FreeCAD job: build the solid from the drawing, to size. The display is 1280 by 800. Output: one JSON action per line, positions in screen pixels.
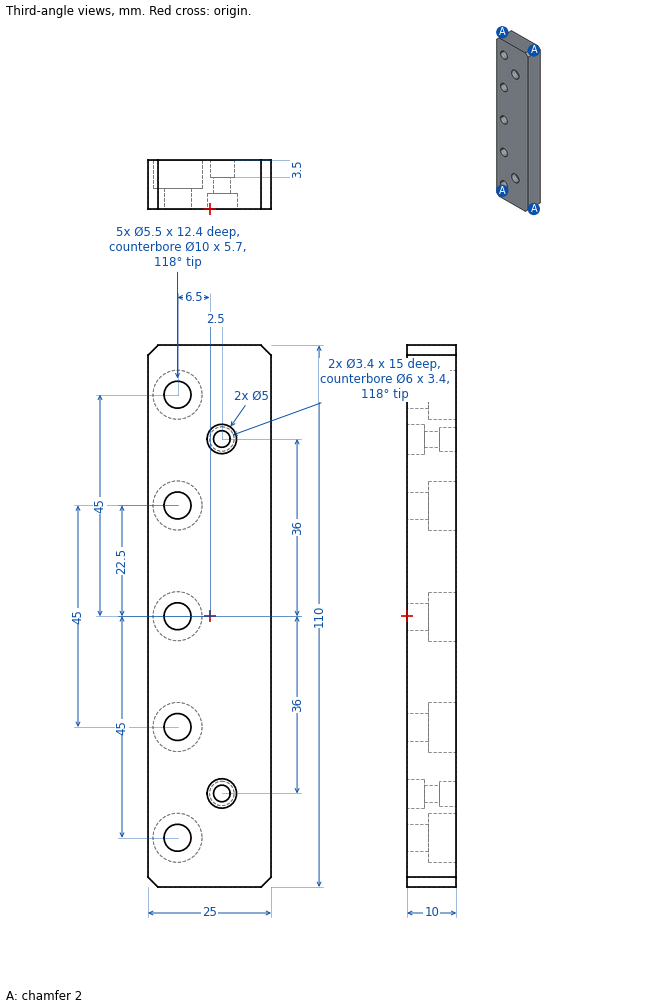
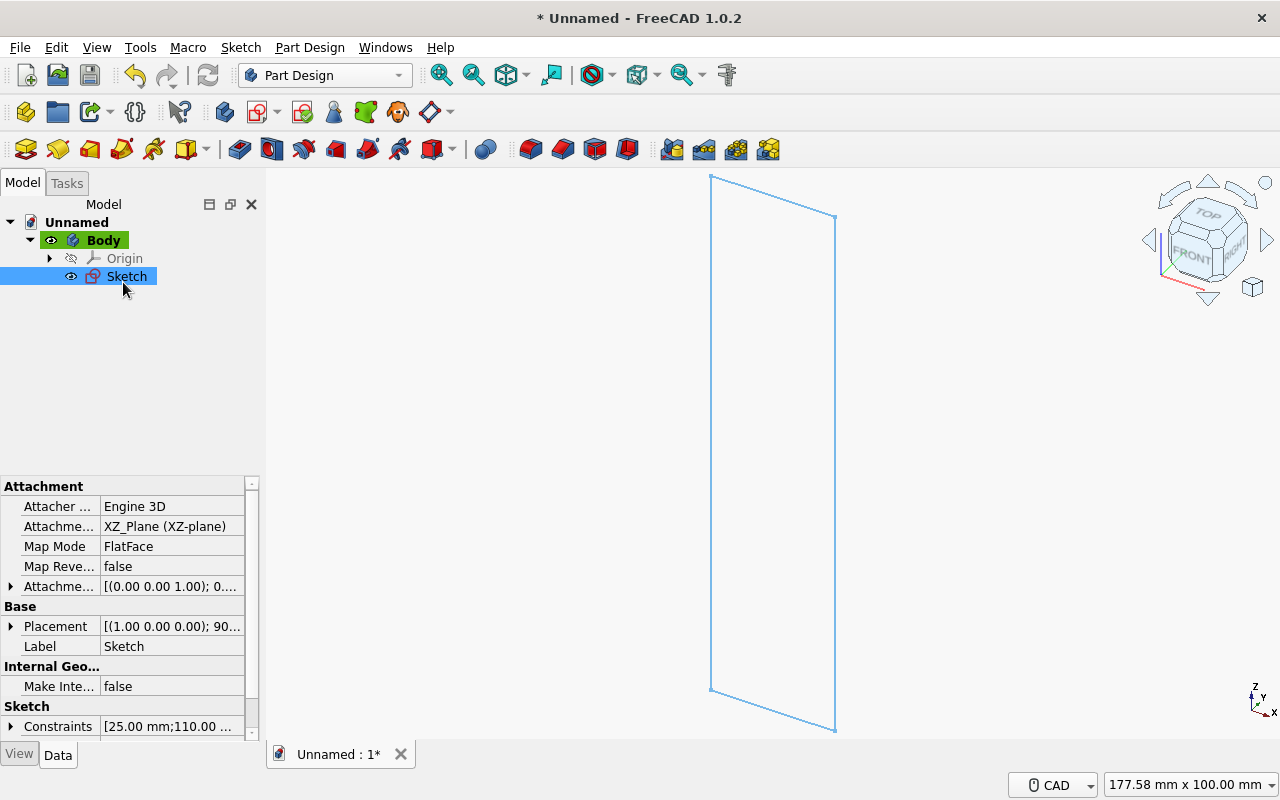
{"action": "left_click", "coordinate": [26, 150]}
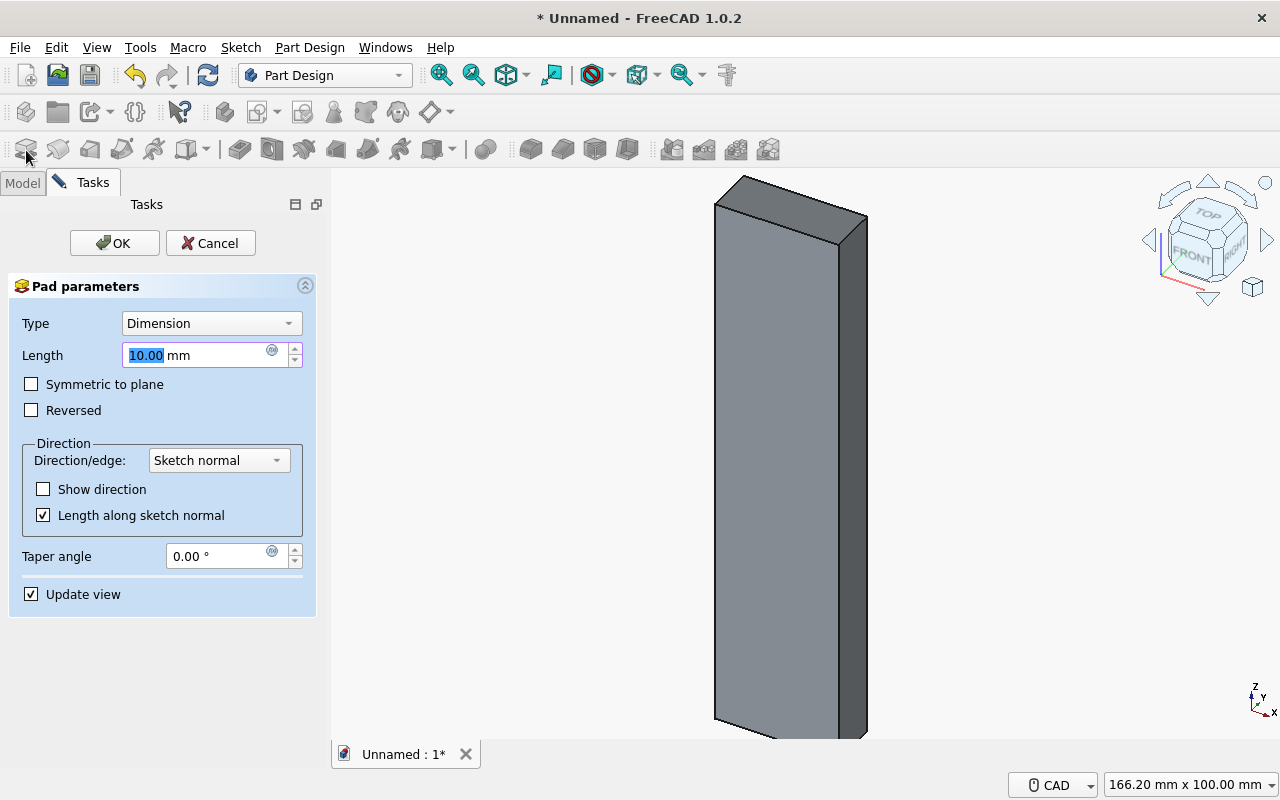
{"action": "type", "text": "10"}
{"action": "key", "text": "Tab"}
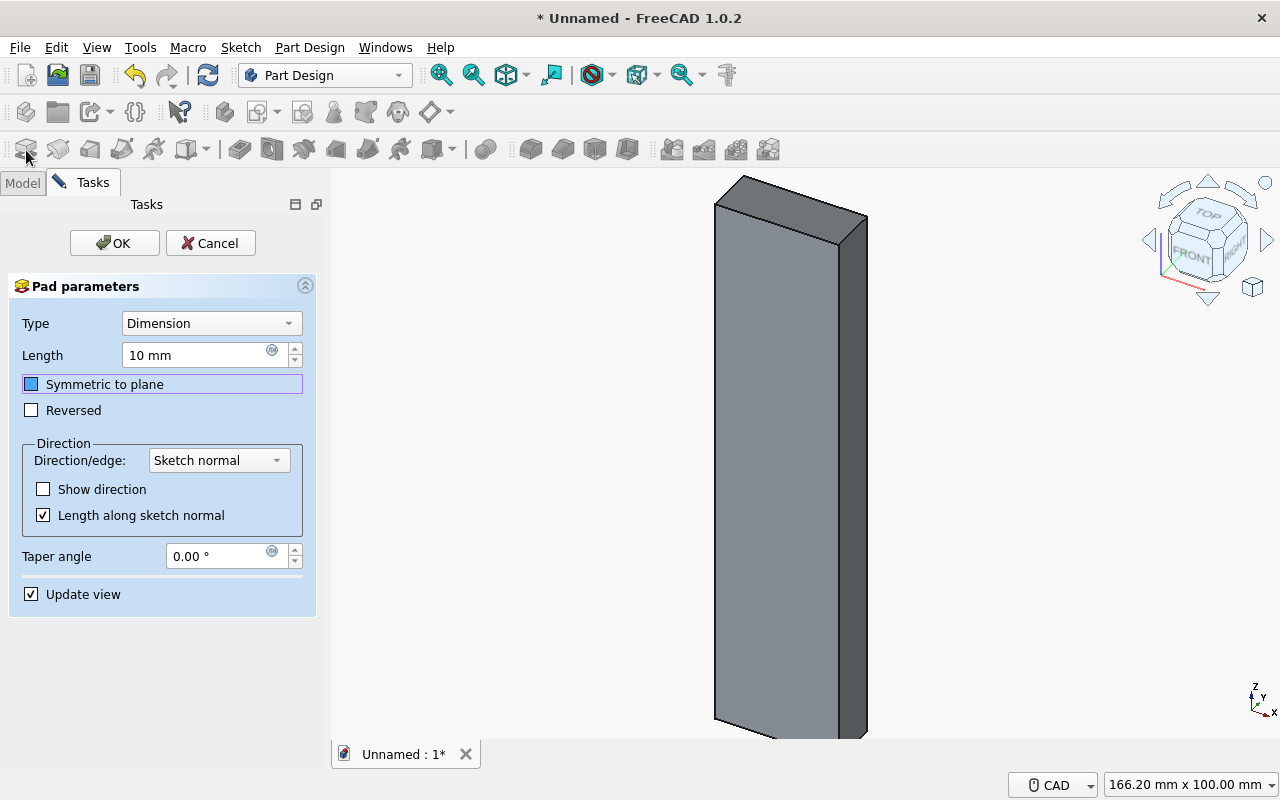
{"action": "left_click", "coordinate": [30, 410]}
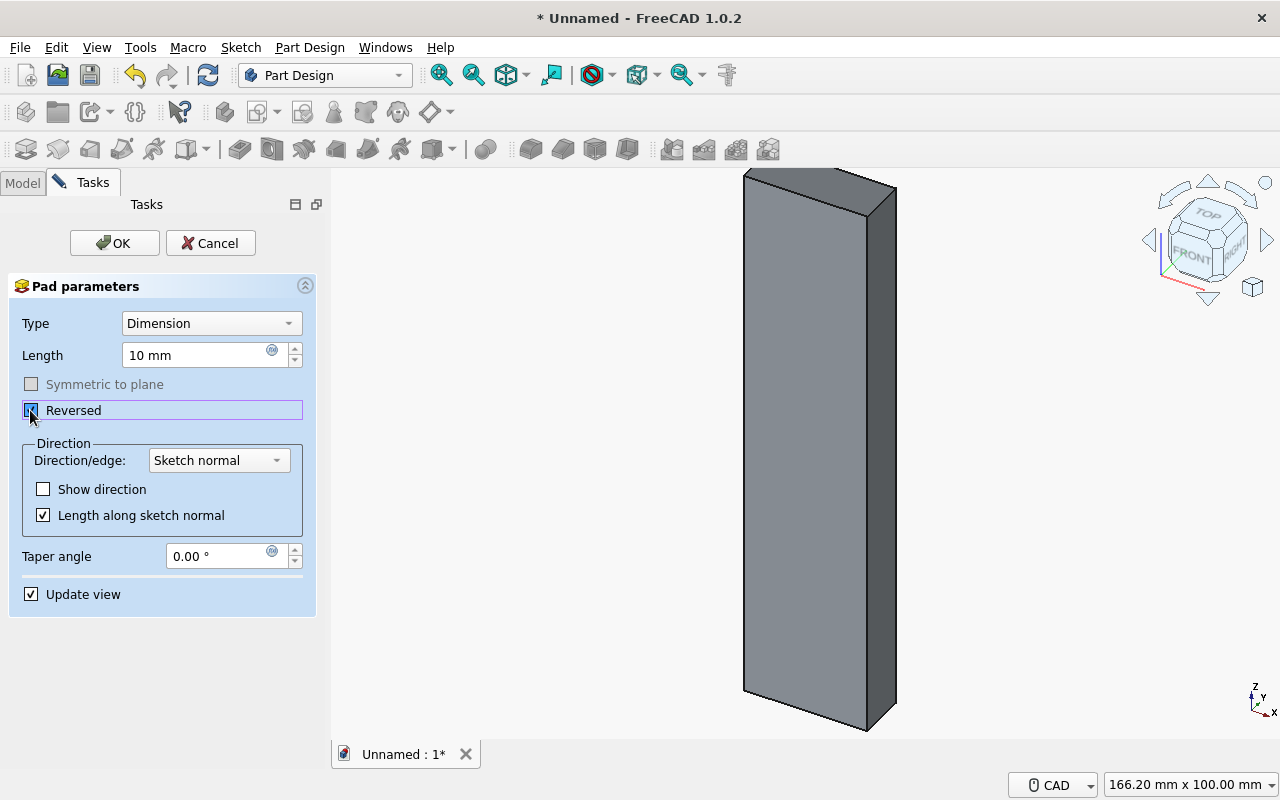
{"action": "left_click", "coordinate": [115, 243]}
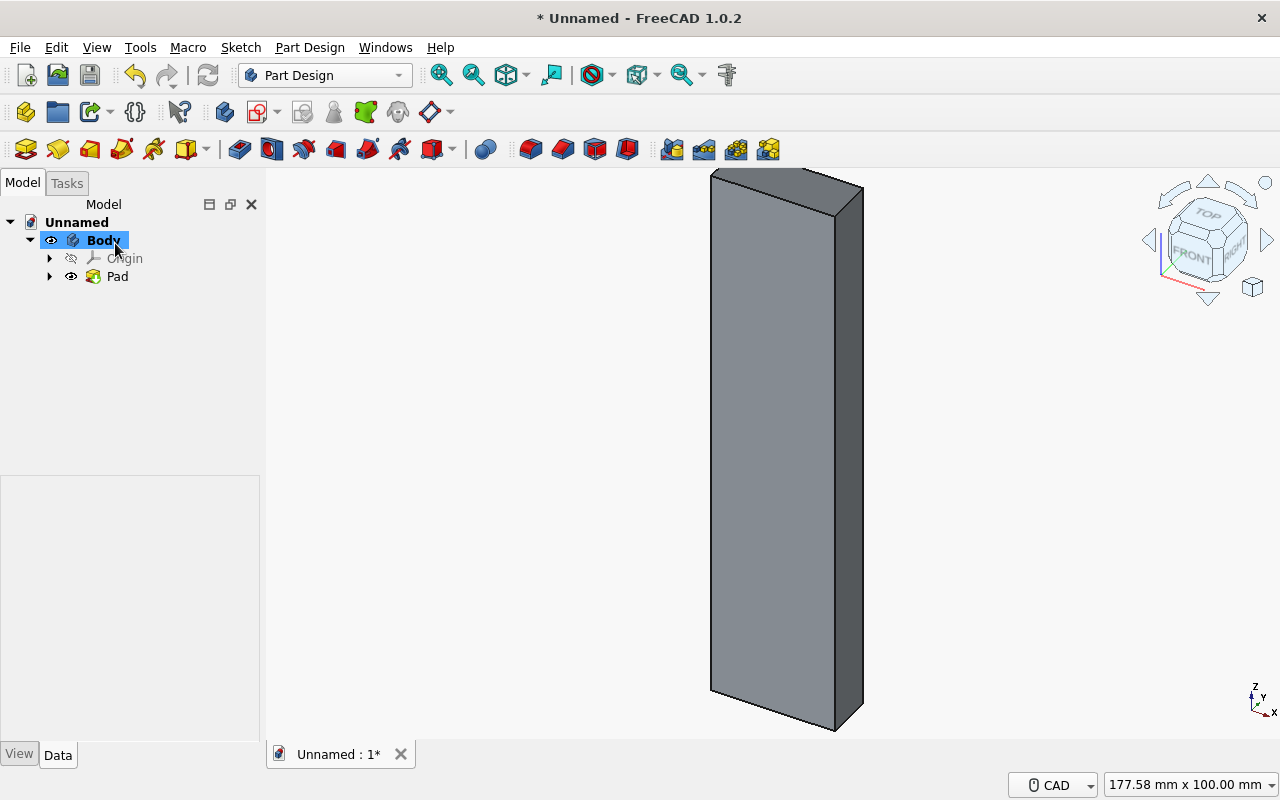
{"action": "left_click", "coordinate": [442, 76]}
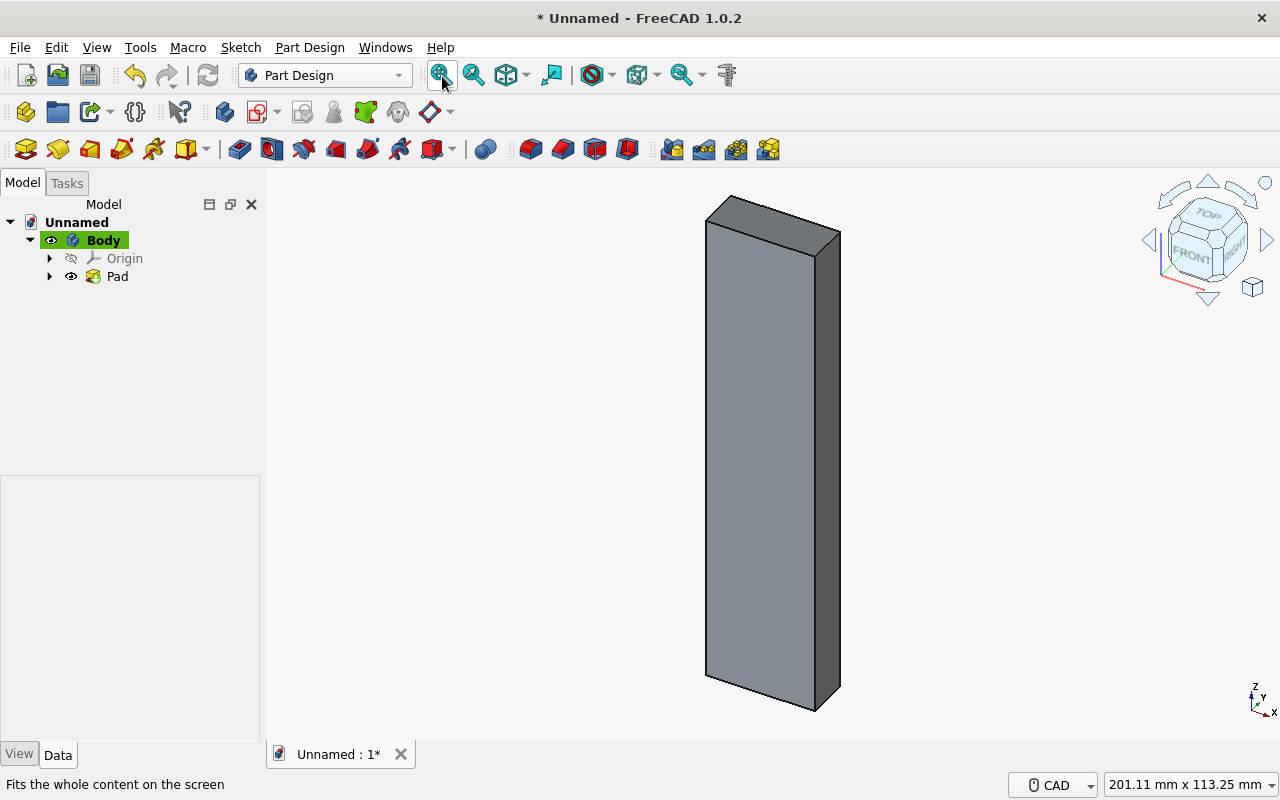
{"action": "left_click", "coordinate": [828, 243]}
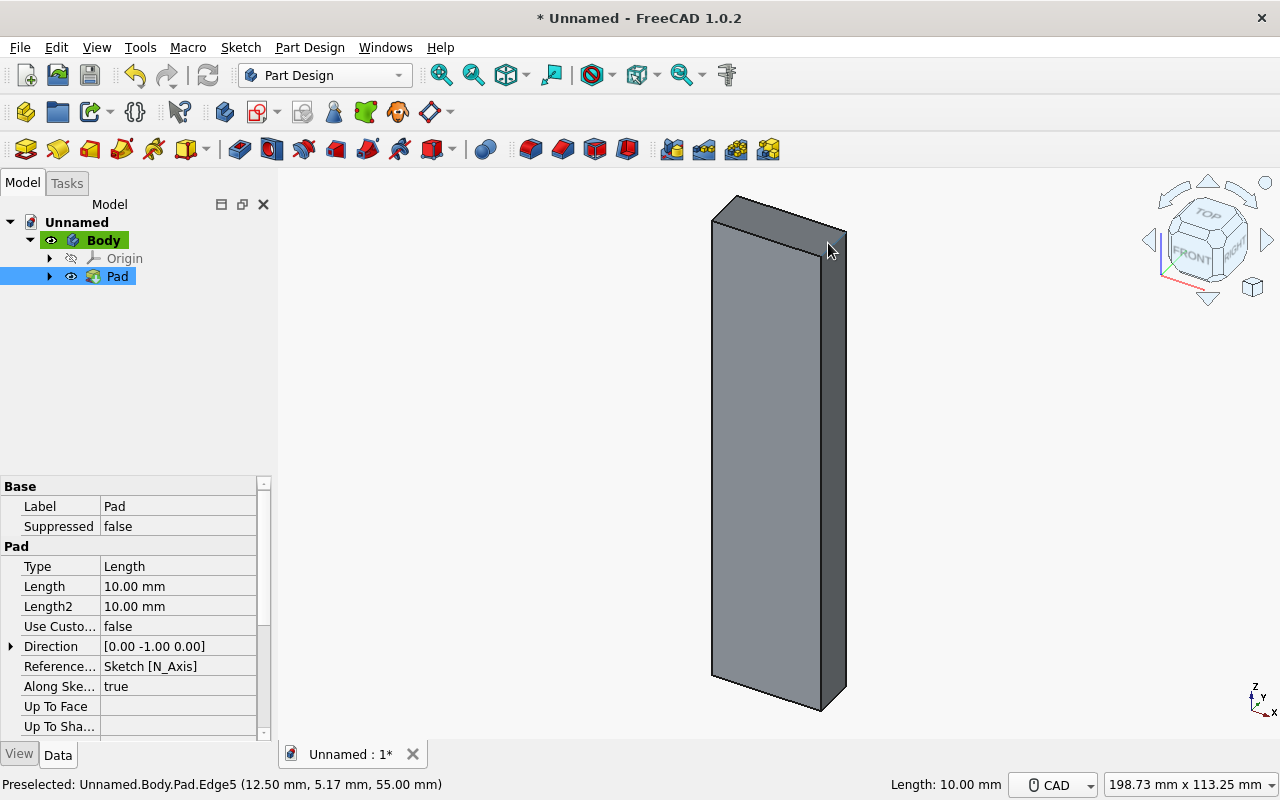
{"action": "key", "text": "0"}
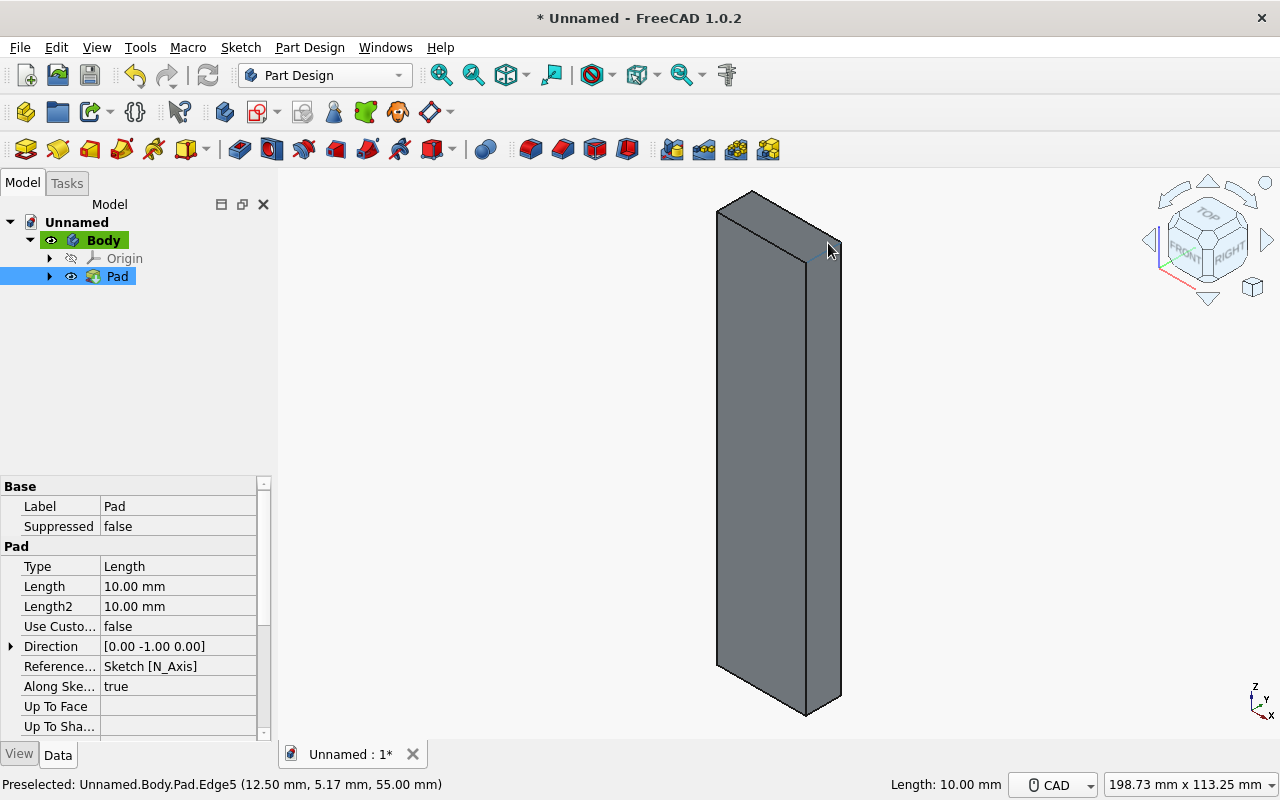
{"action": "key", "text": "2"}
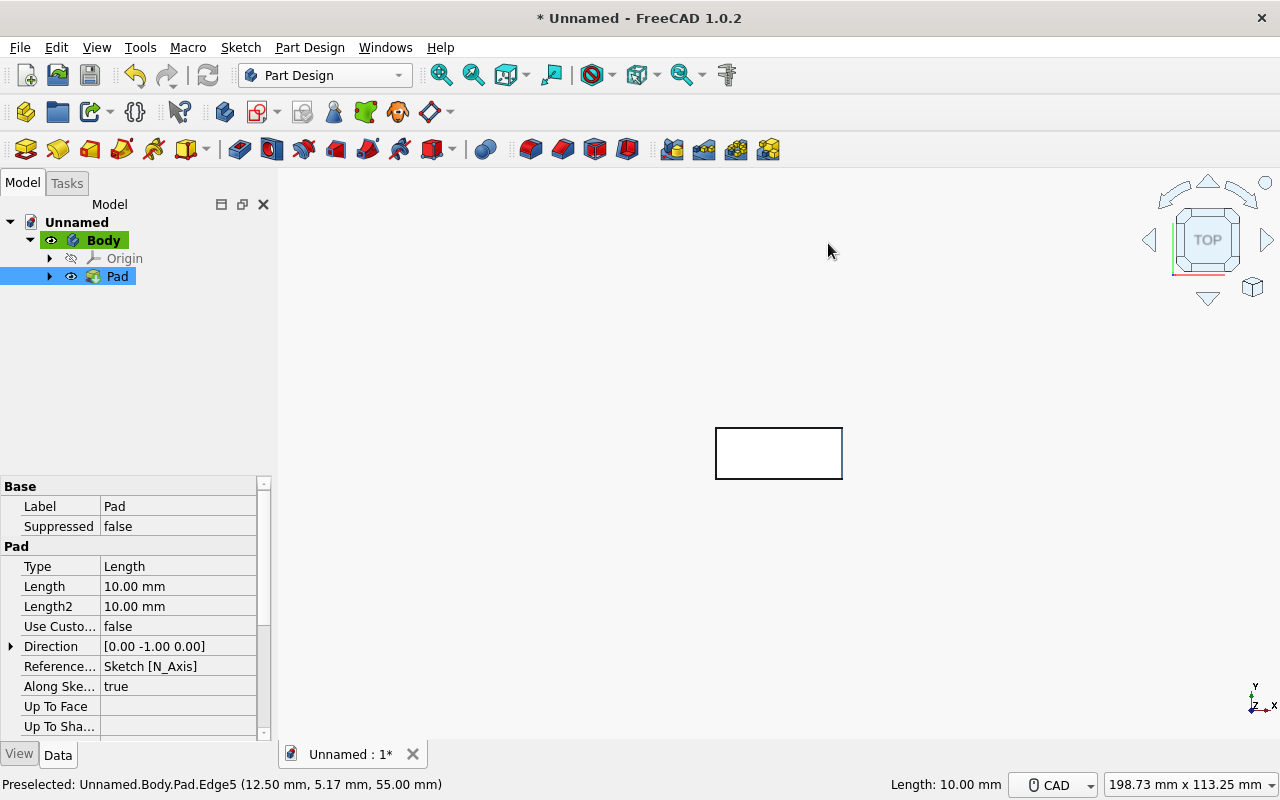
{"action": "left_click", "coordinate": [442, 76]}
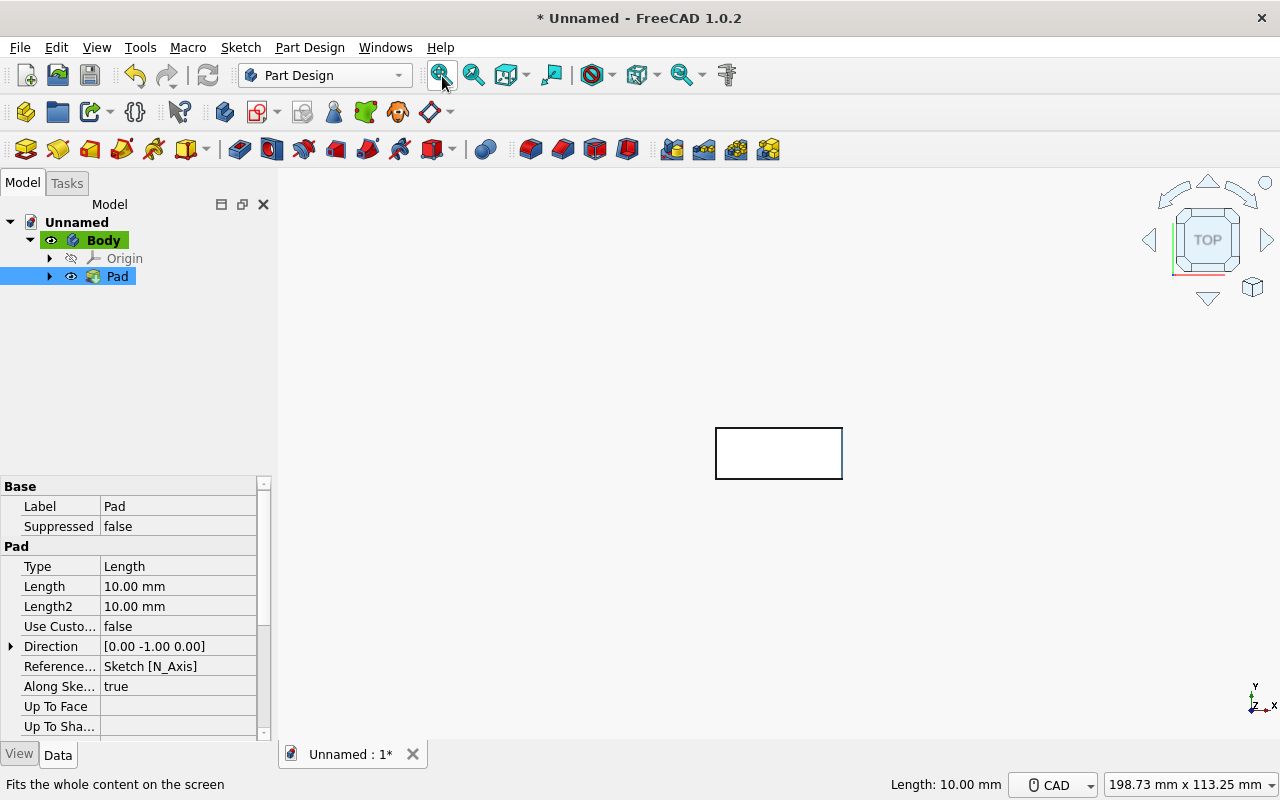
{"action": "left_click", "coordinate": [716, 452], "text": "ctrl"}